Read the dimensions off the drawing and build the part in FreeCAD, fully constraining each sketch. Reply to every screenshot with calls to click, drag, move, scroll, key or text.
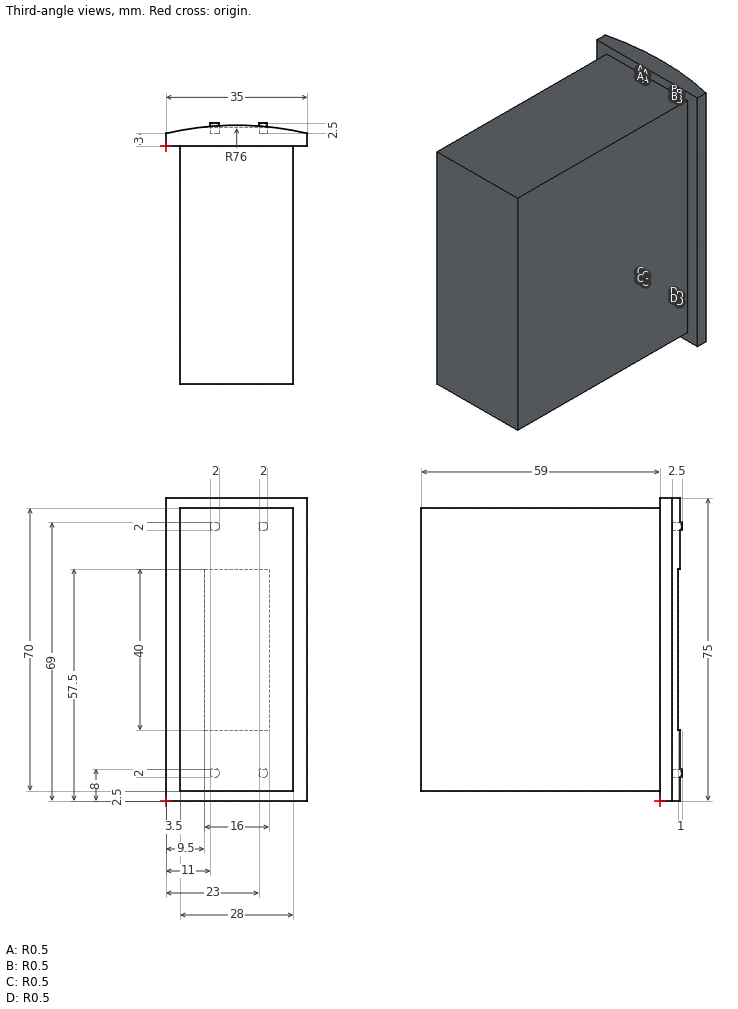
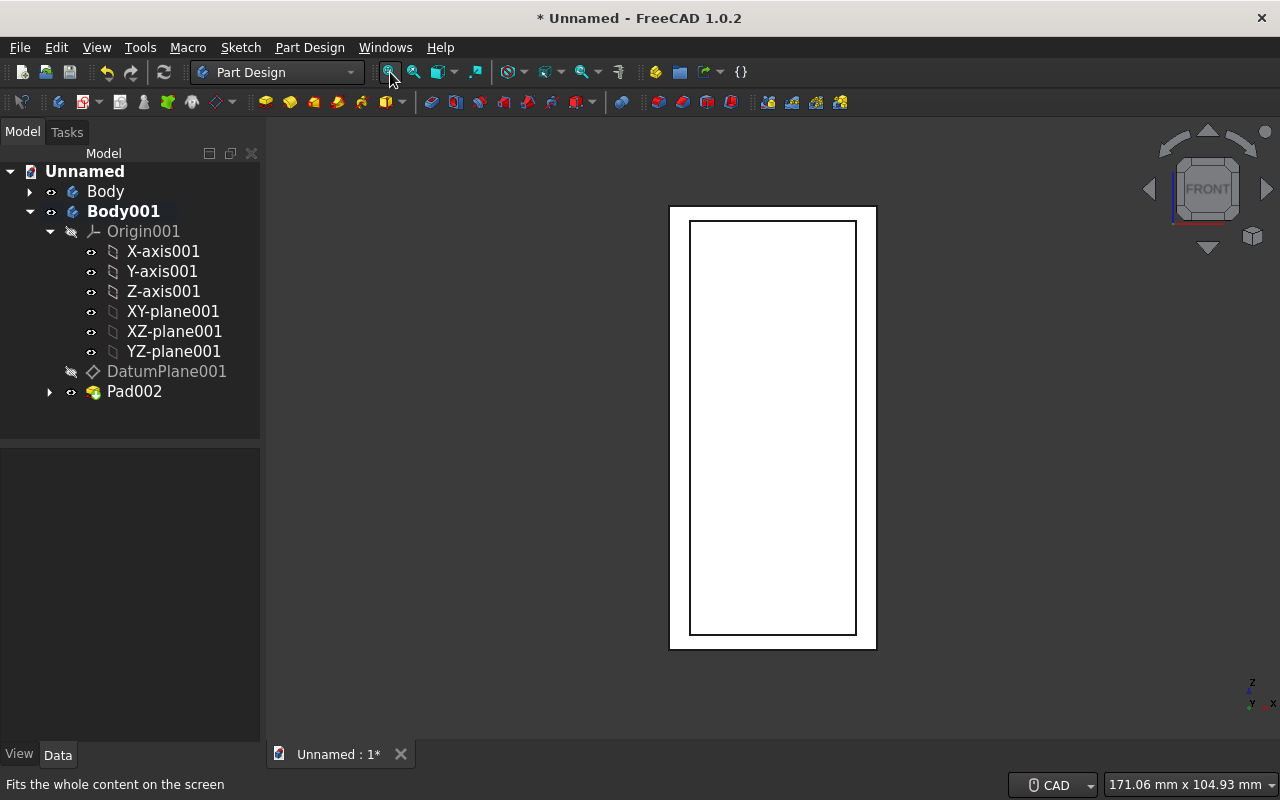
key(3)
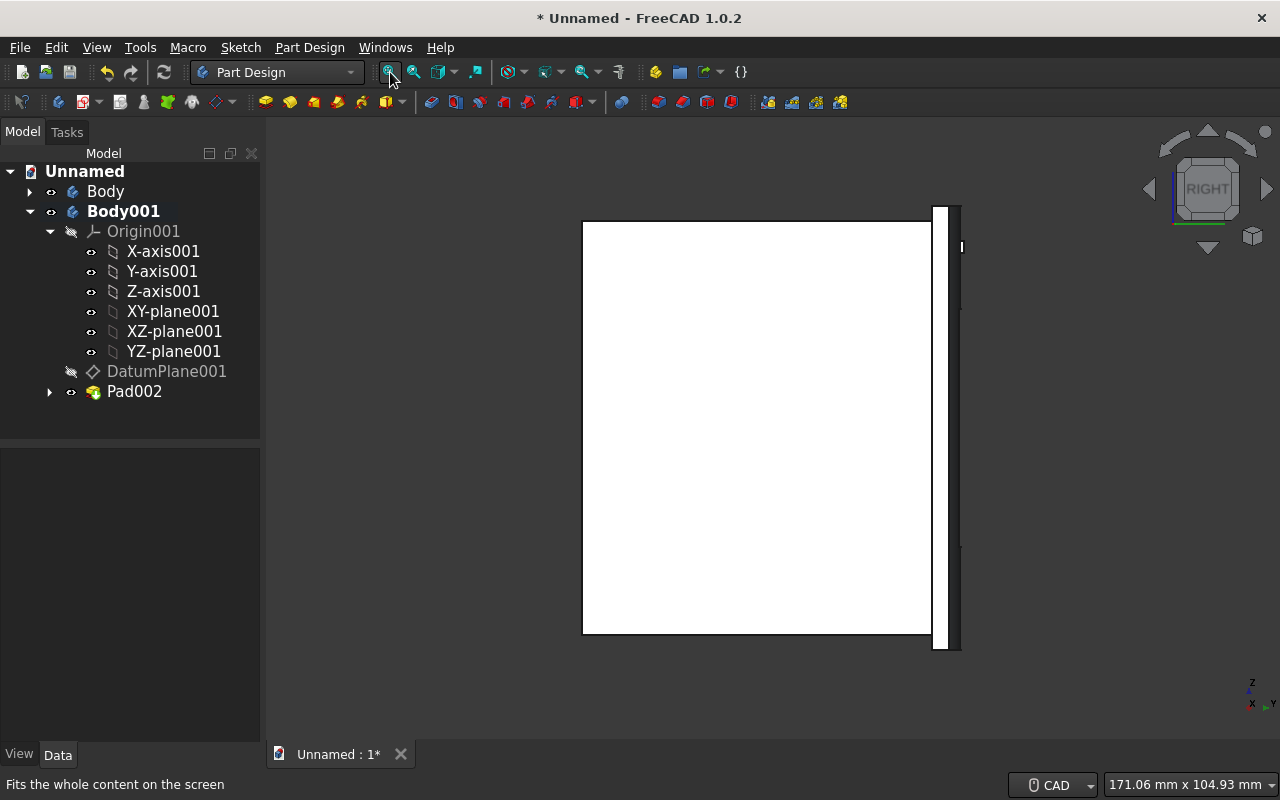
key(v)
key(f)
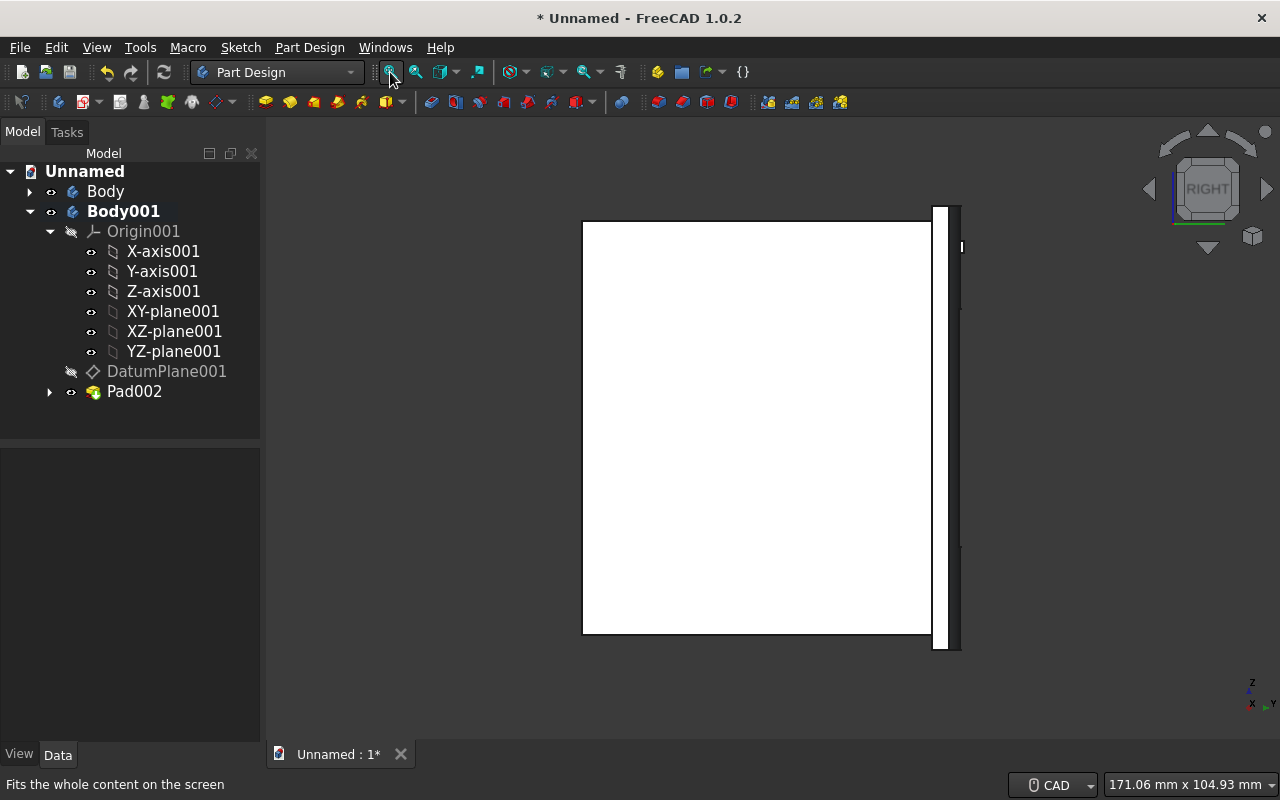
scroll(957, 240, up, 5)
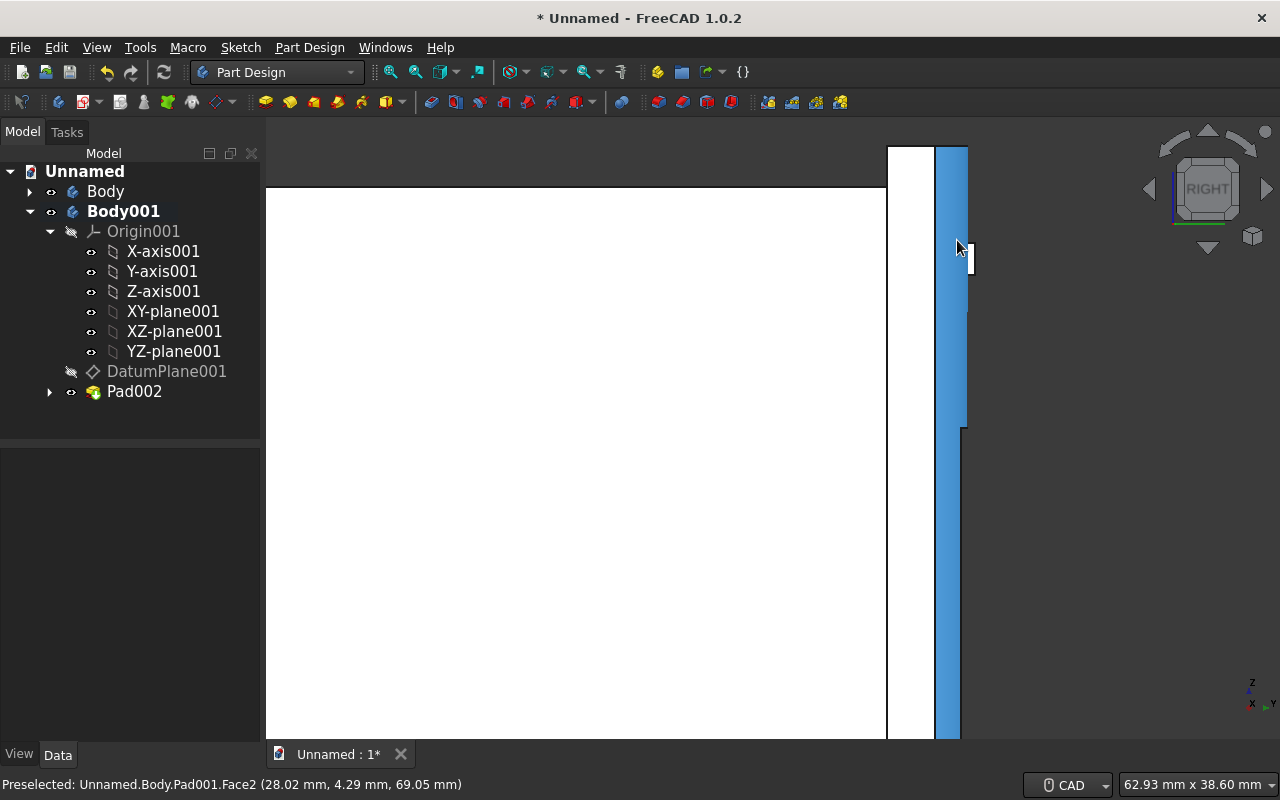
key(v)
key(f)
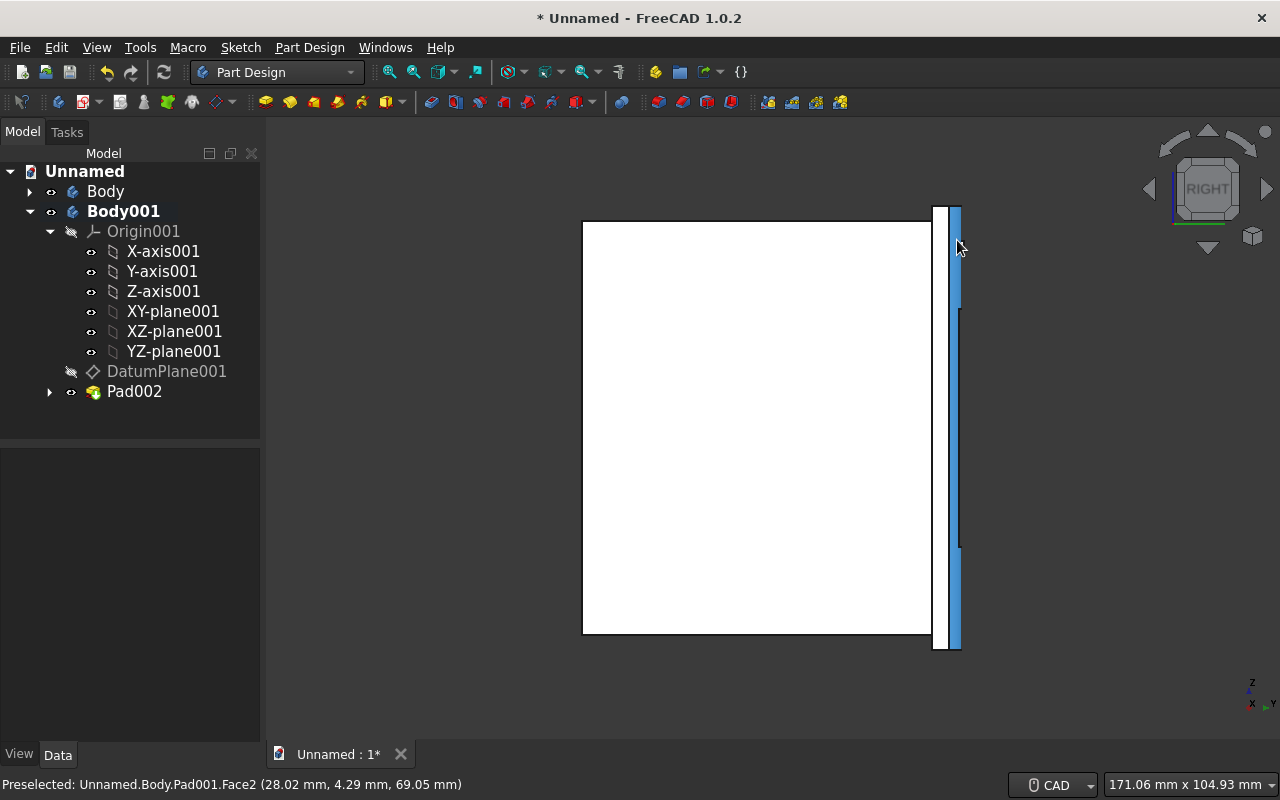
key(5)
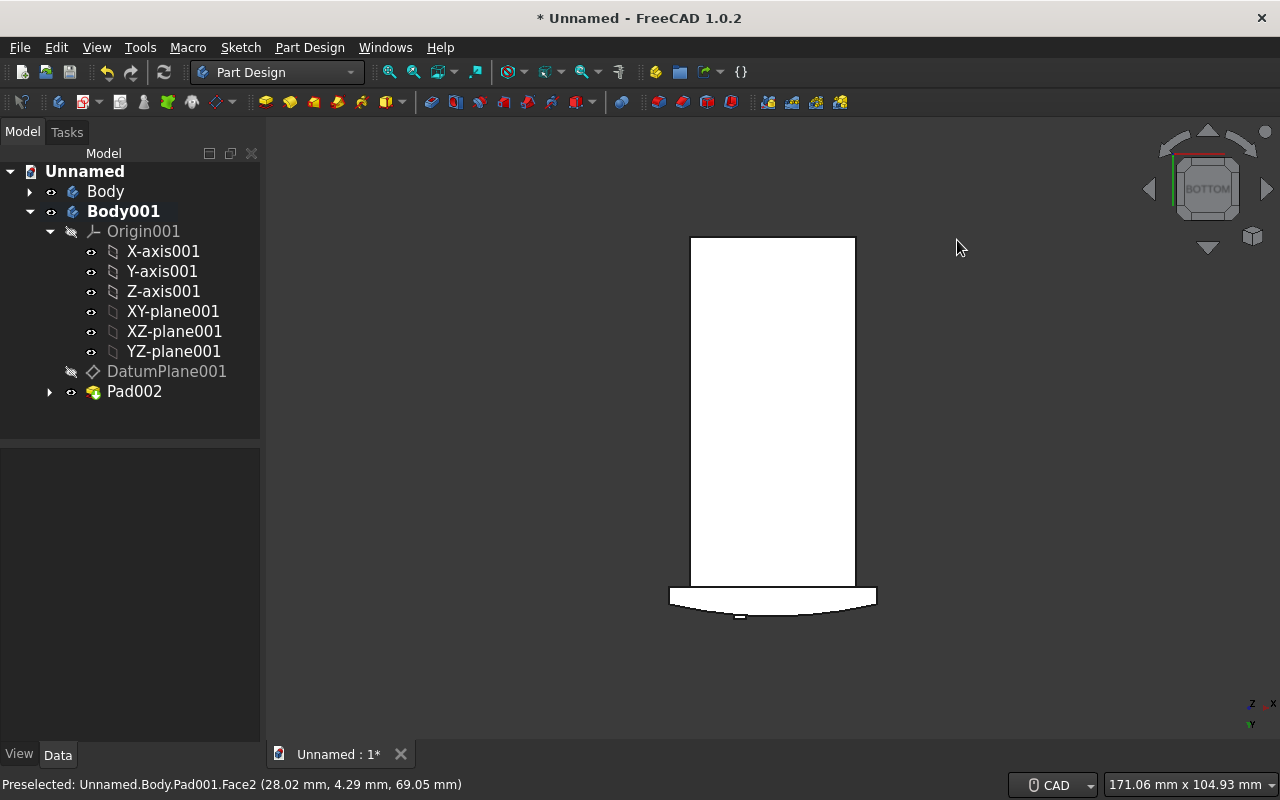
key(v)
key(f)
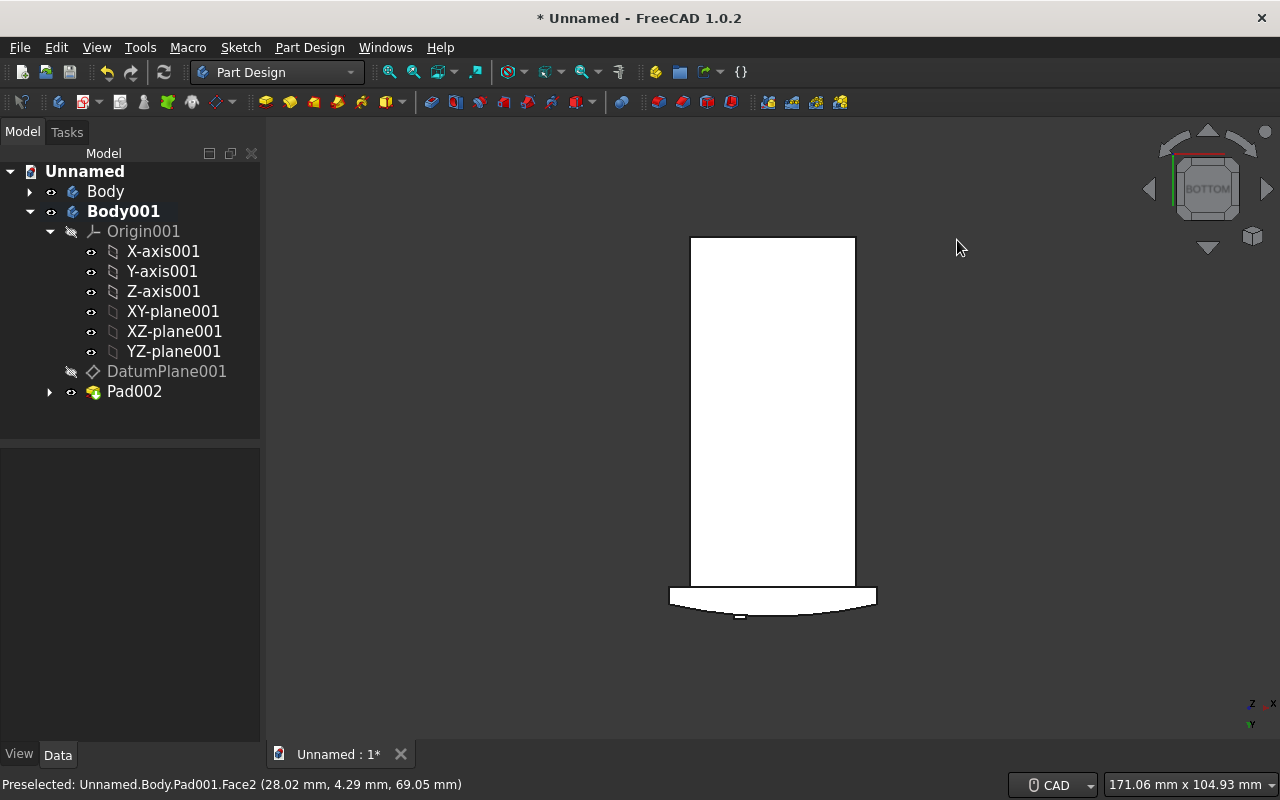
scroll(734, 611, up, 5)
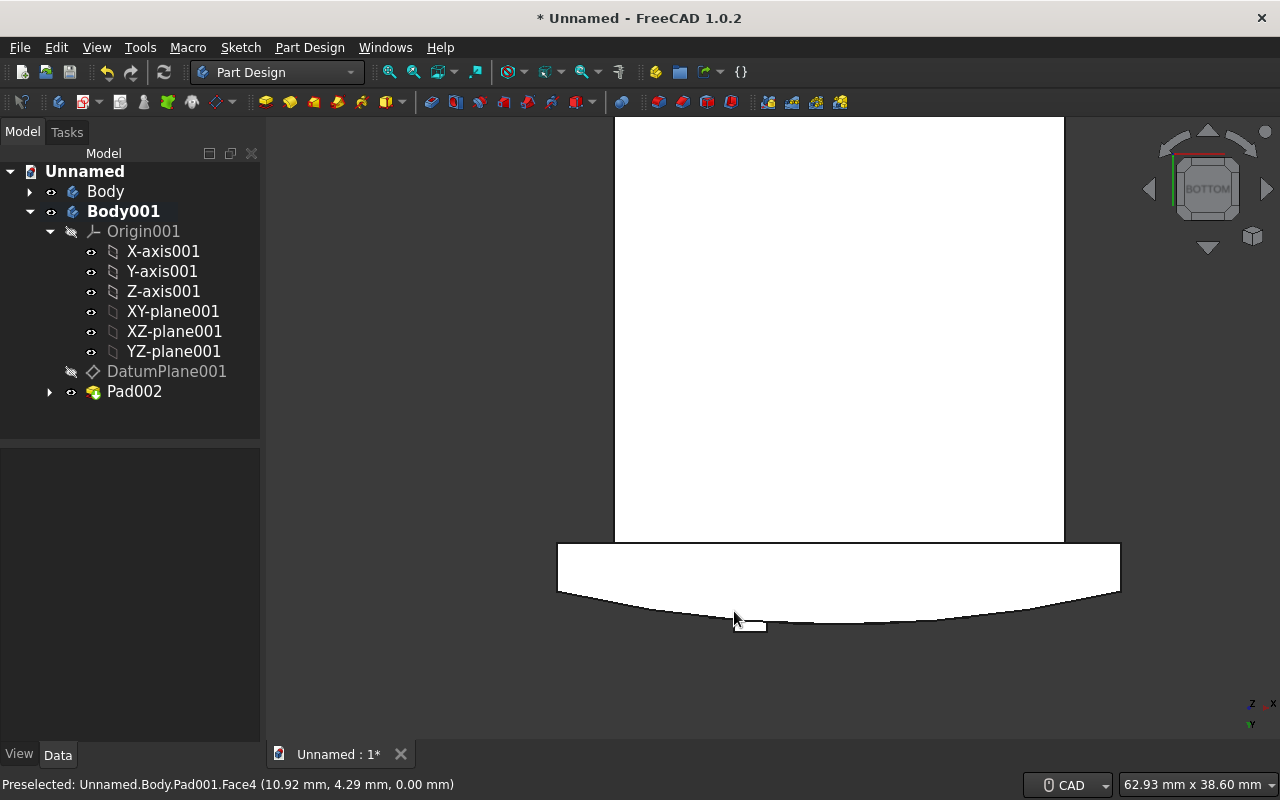
key(v)
key(f)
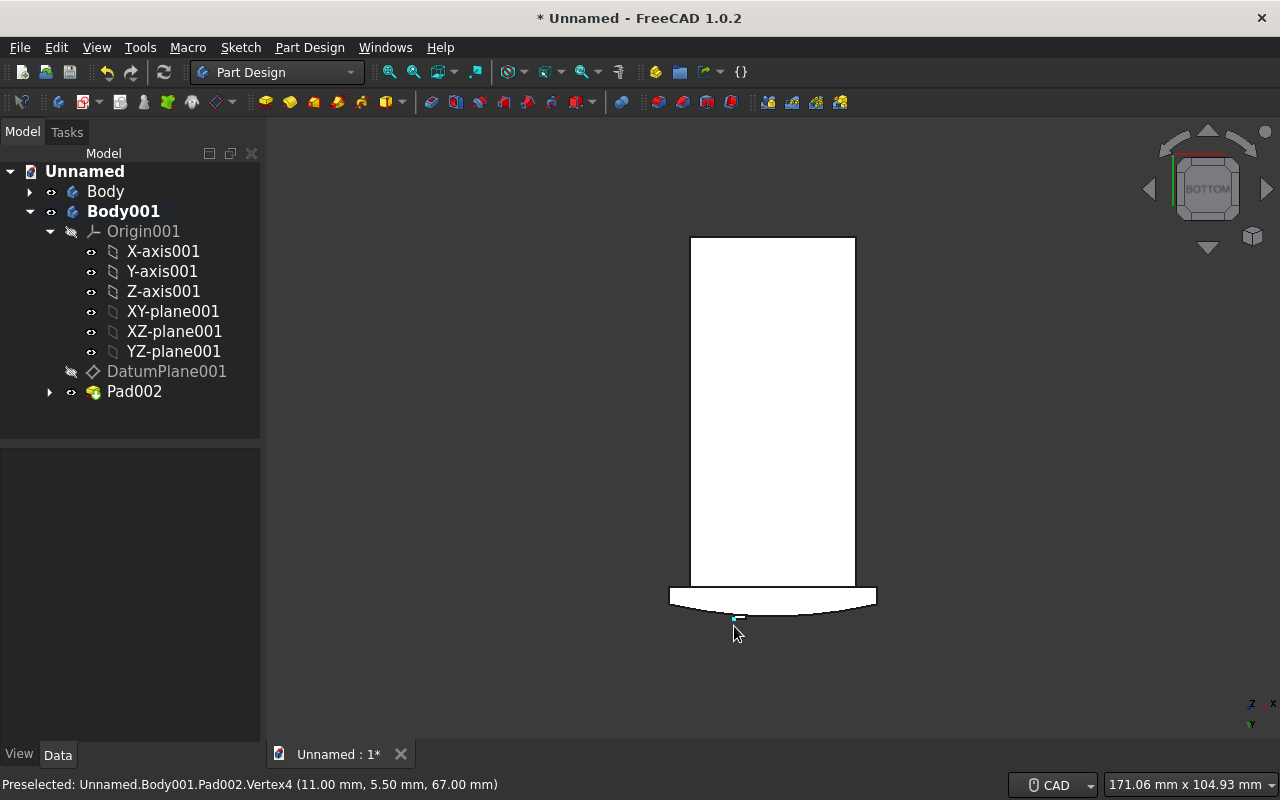
key(4)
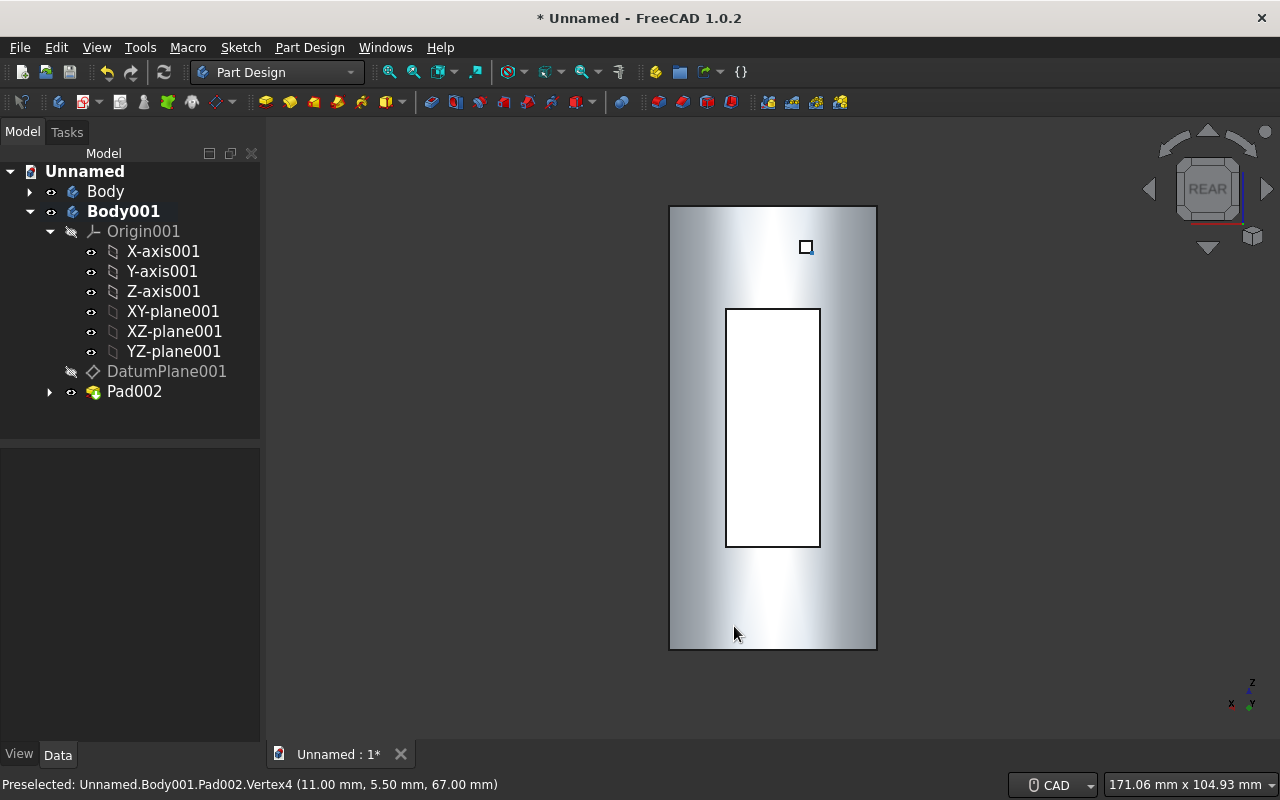
key(v)
key(f)